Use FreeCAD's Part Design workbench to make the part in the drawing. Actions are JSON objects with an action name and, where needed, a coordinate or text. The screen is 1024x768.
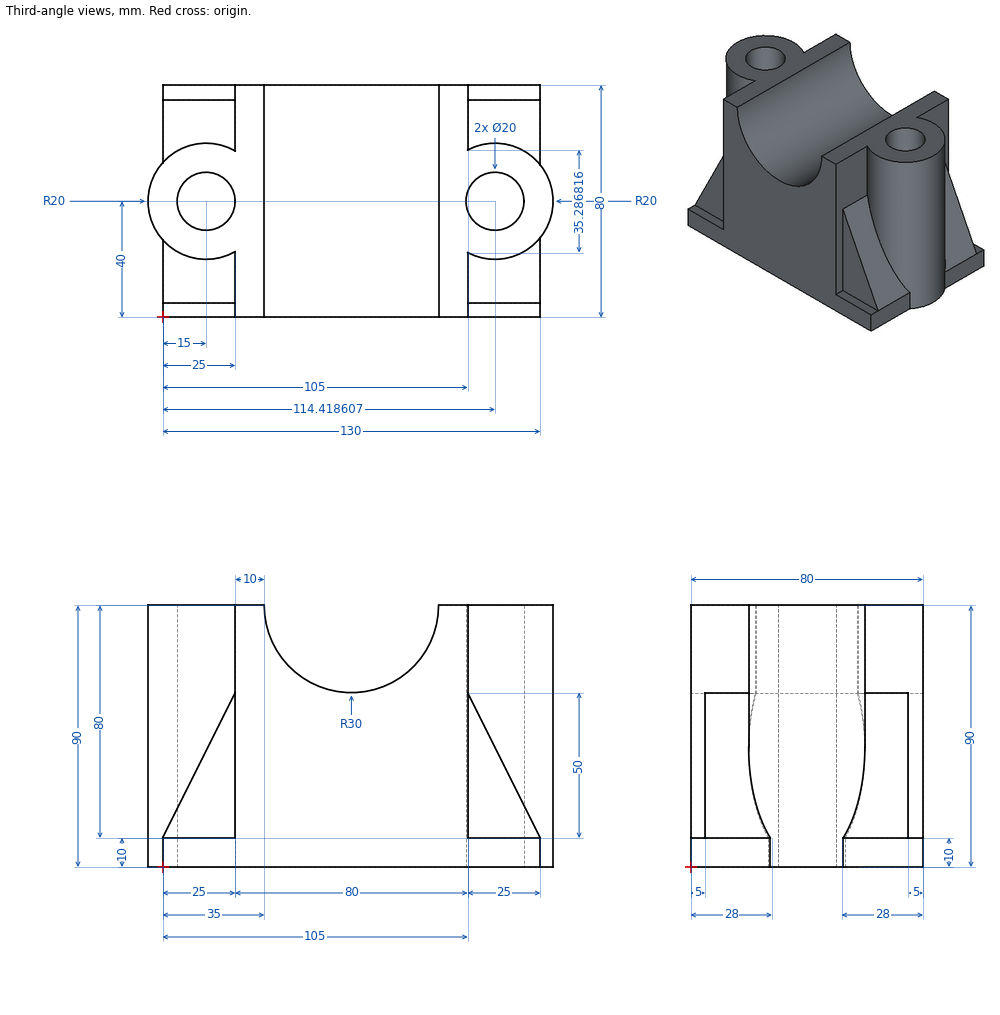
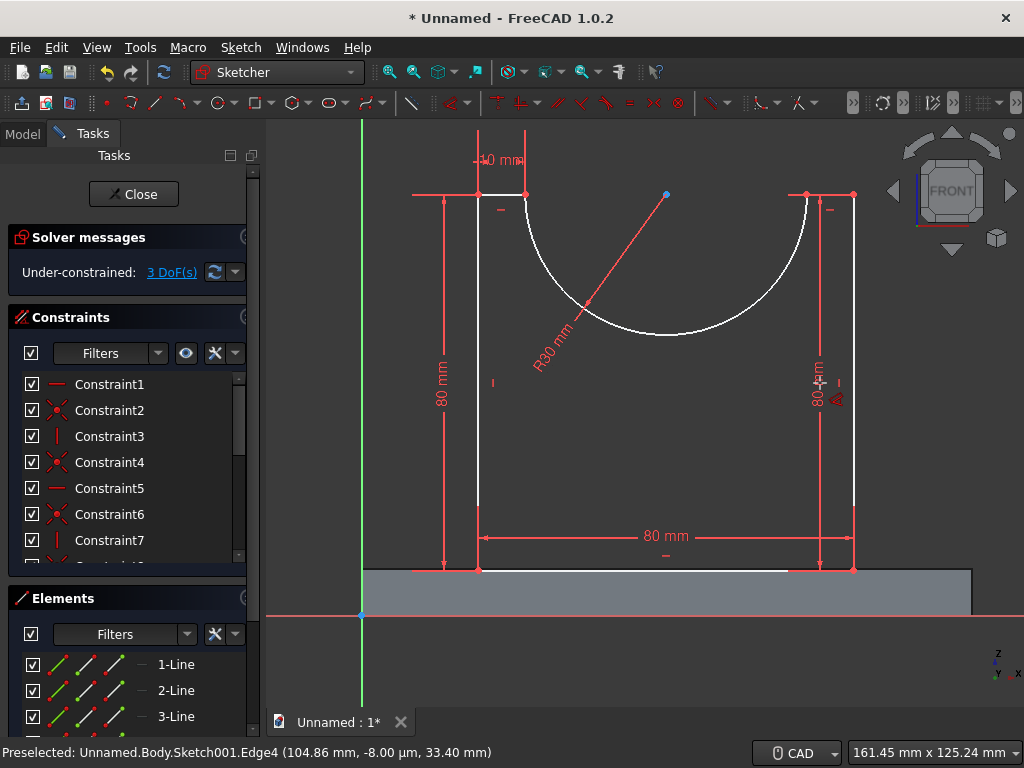
{"action": "left_click", "coordinate": [525, 195]}
{"action": "left_click", "coordinate": [443, 650]}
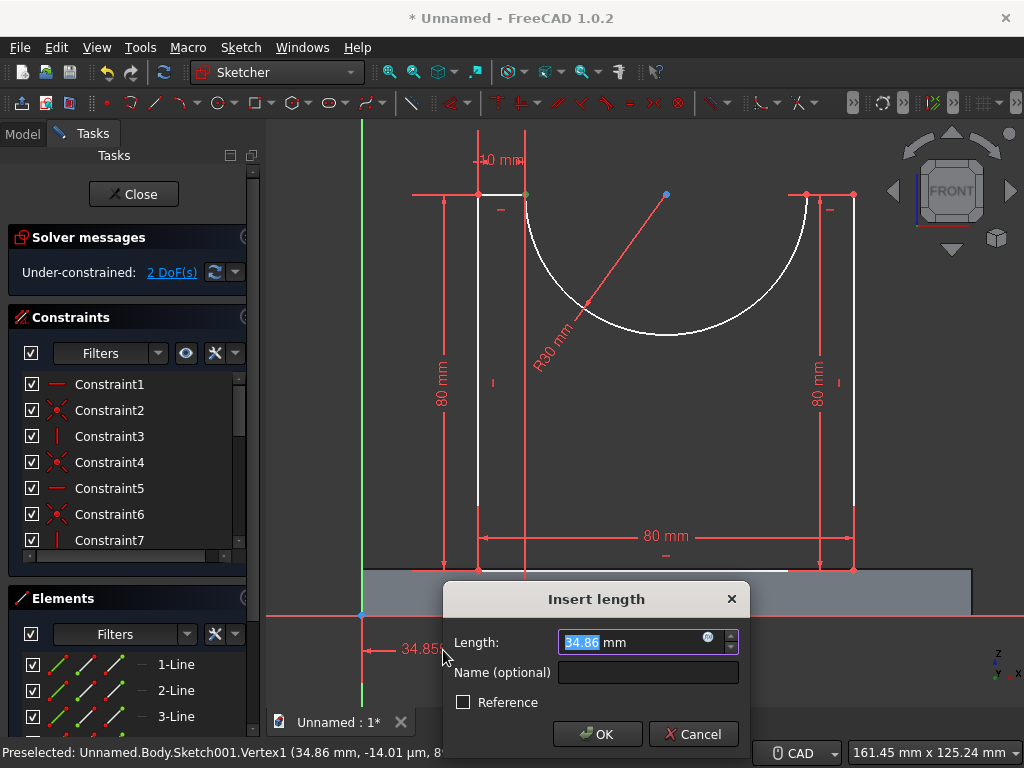
{"action": "type", "text": "35"}
{"action": "key", "text": "Return"}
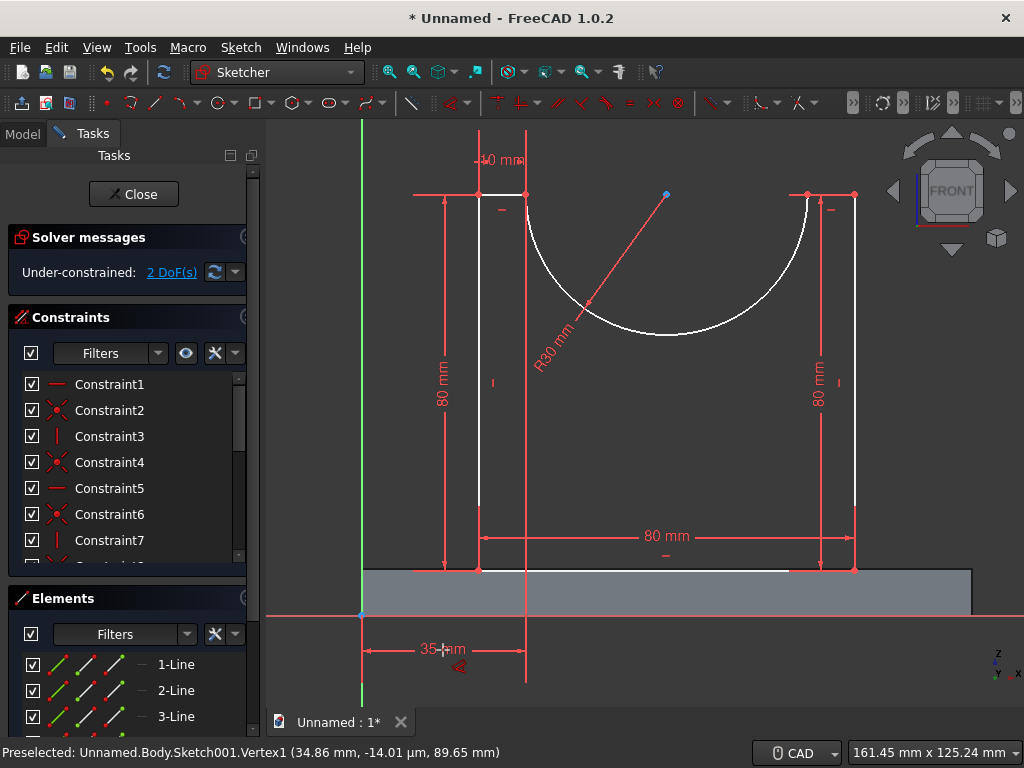
{"action": "left_click", "coordinate": [526, 195]}
{"action": "left_click", "coordinate": [328, 405]}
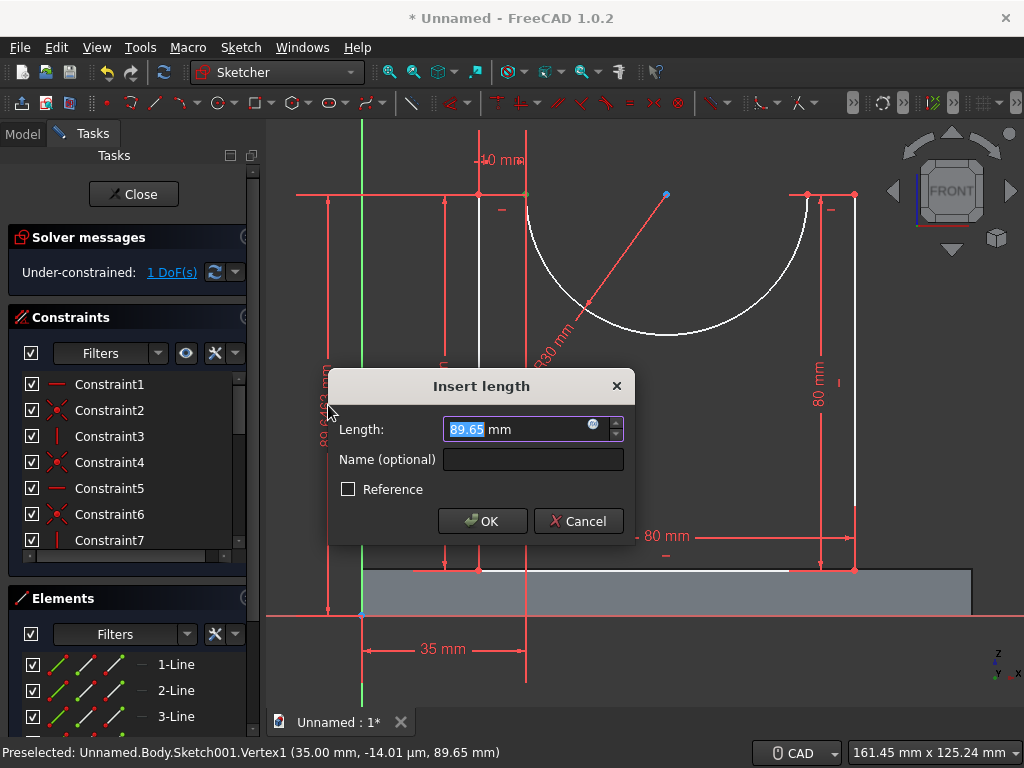
{"action": "type", "text": "90"}
{"action": "key", "text": "Return"}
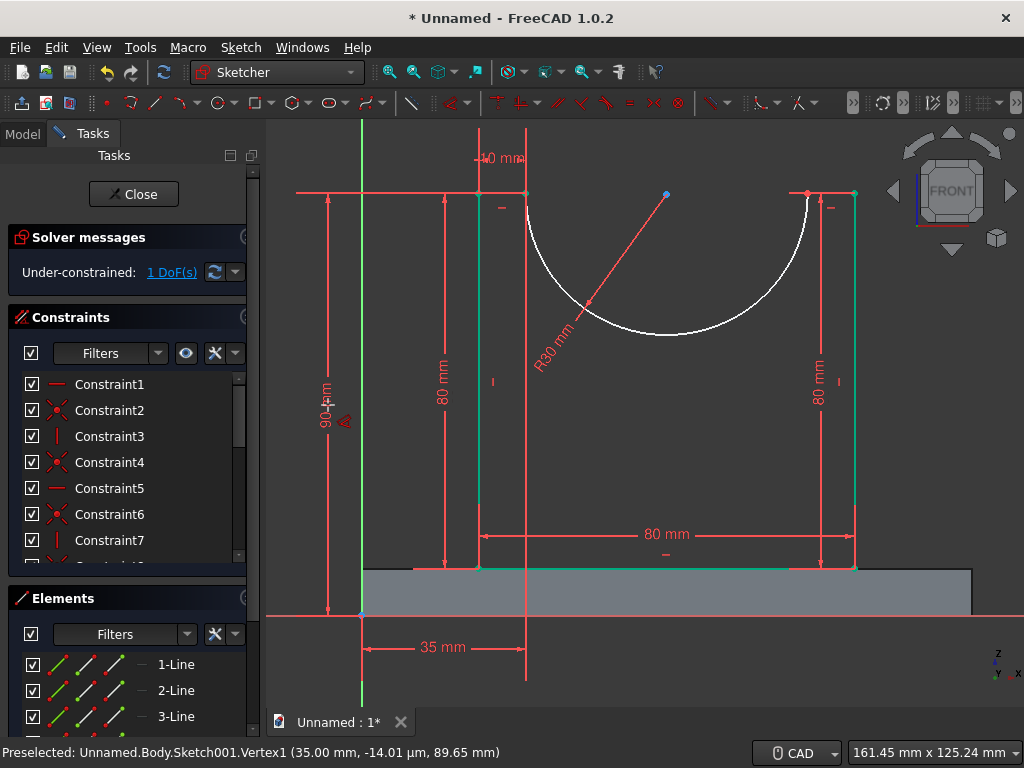
{"action": "left_click", "coordinate": [667, 194]}
{"action": "left_click", "coordinate": [328, 308]}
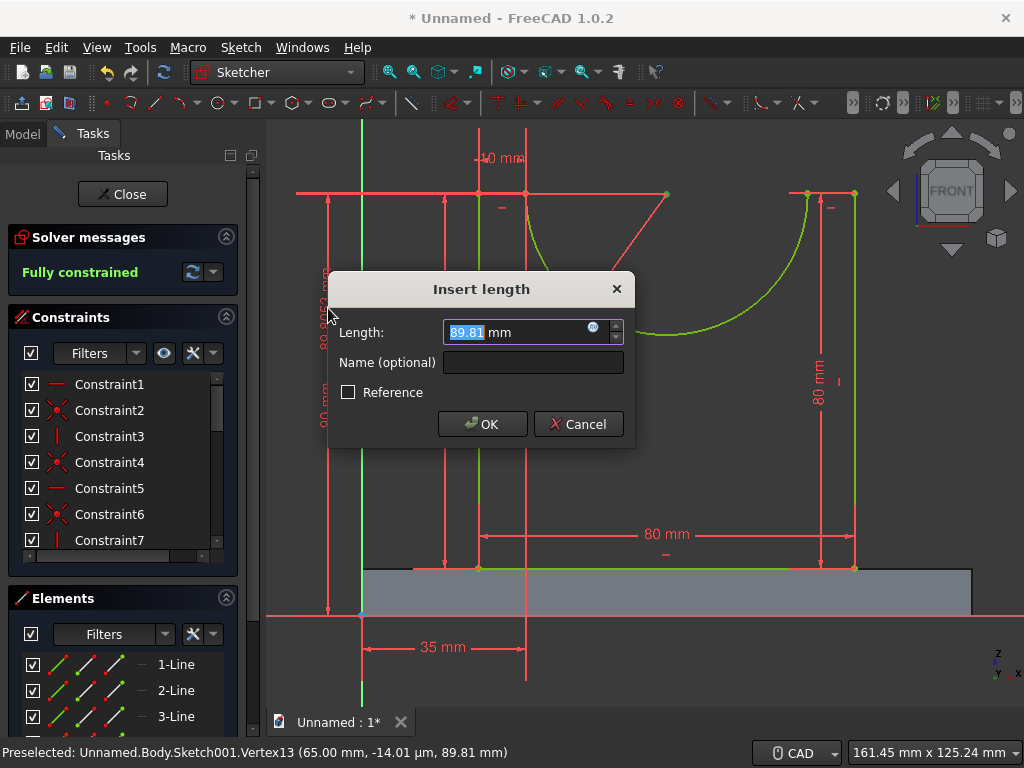
{"action": "type", "text": "90"}
{"action": "key", "text": "Return"}
{"action": "key", "text": "Escape"}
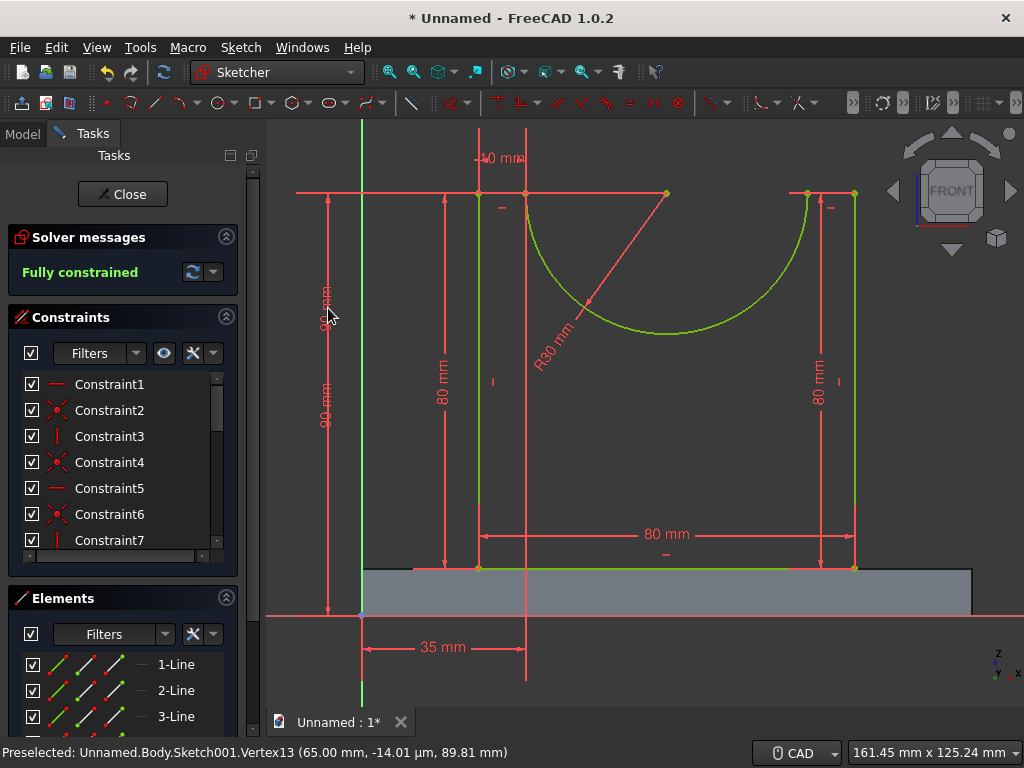
{"action": "left_click", "coordinate": [123, 194]}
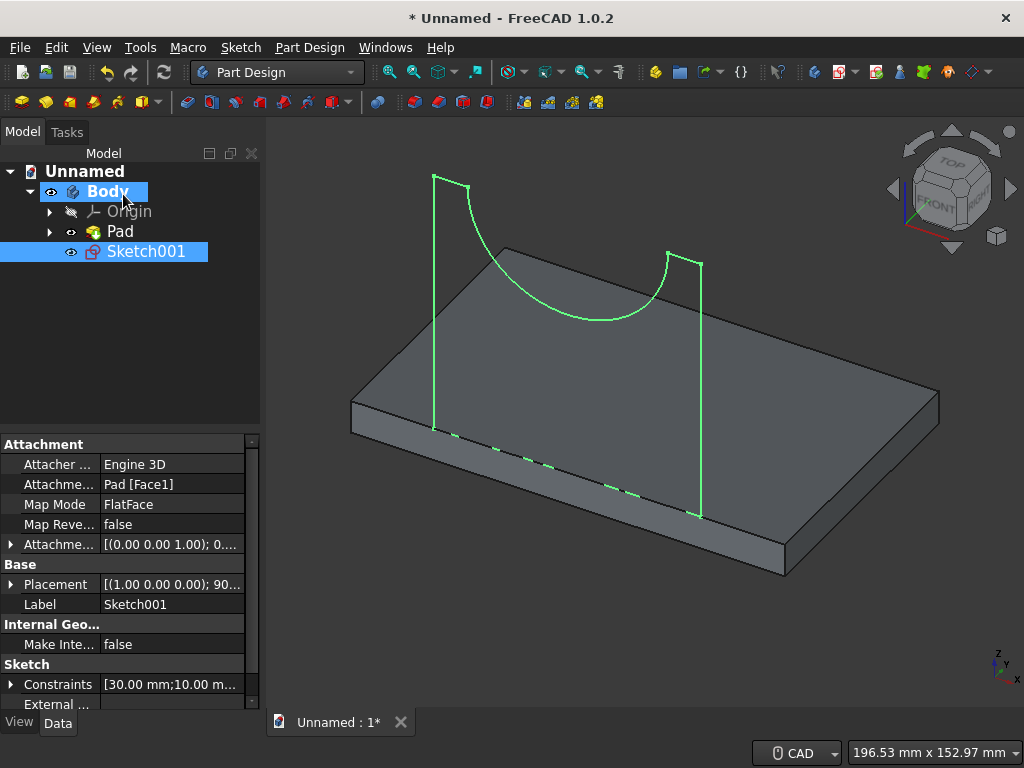
{"action": "left_click", "coordinate": [22, 102]}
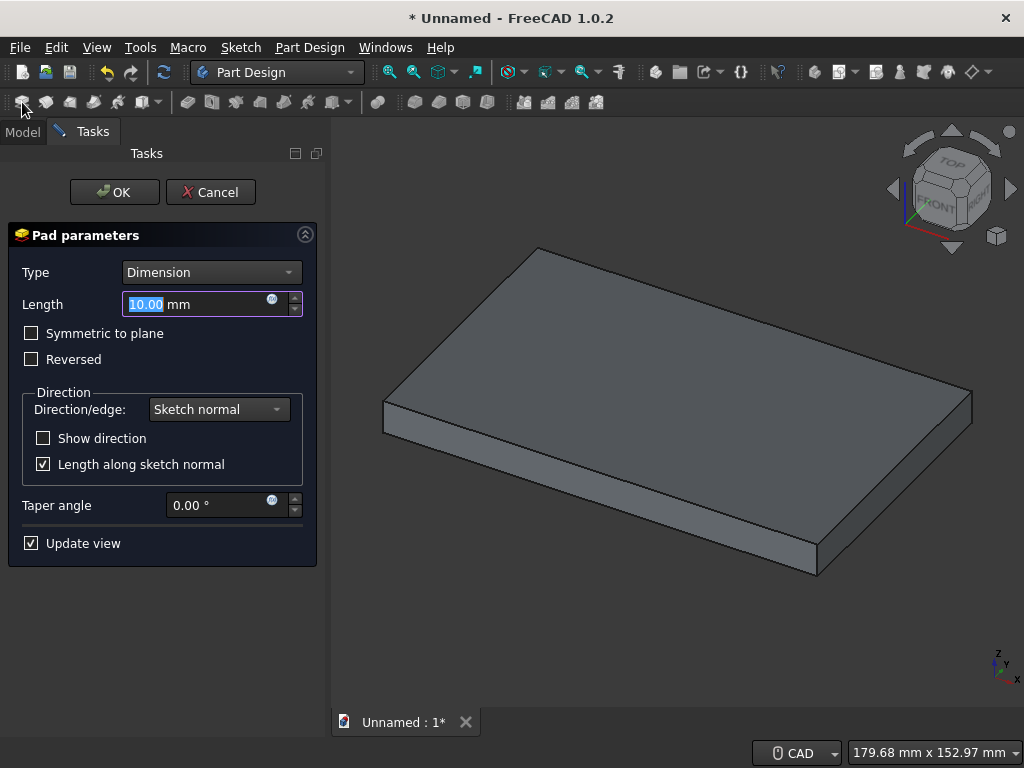
{"action": "type", "text": "80"}
{"action": "key", "text": "Tab"}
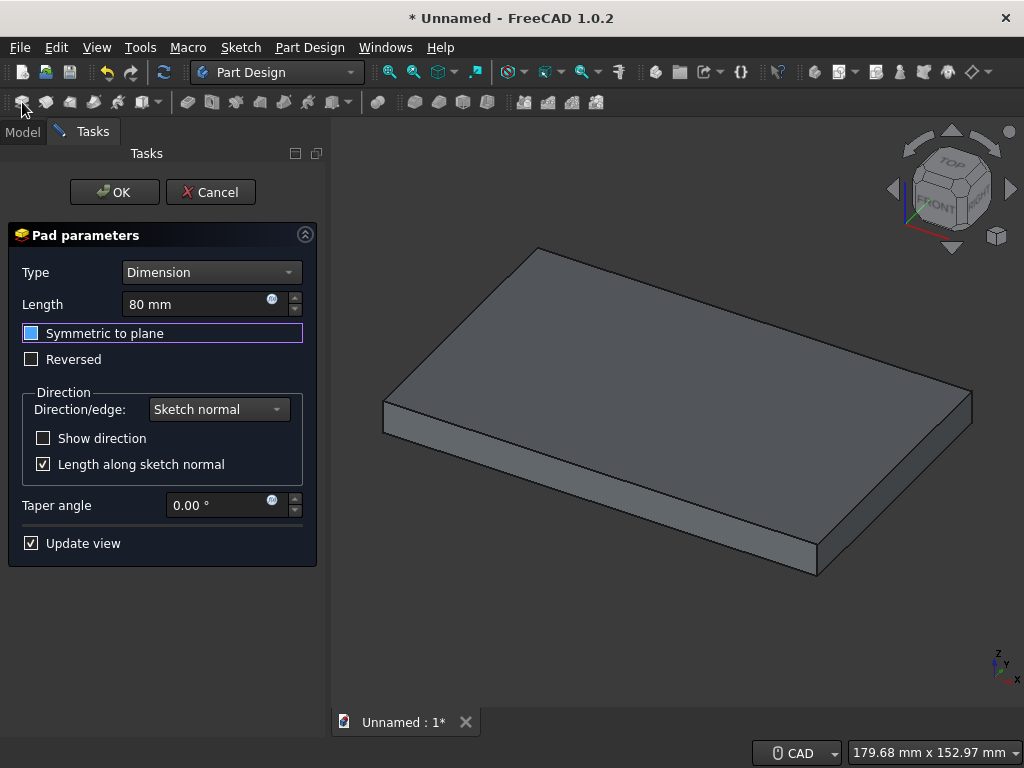
{"action": "left_click", "coordinate": [30, 359]}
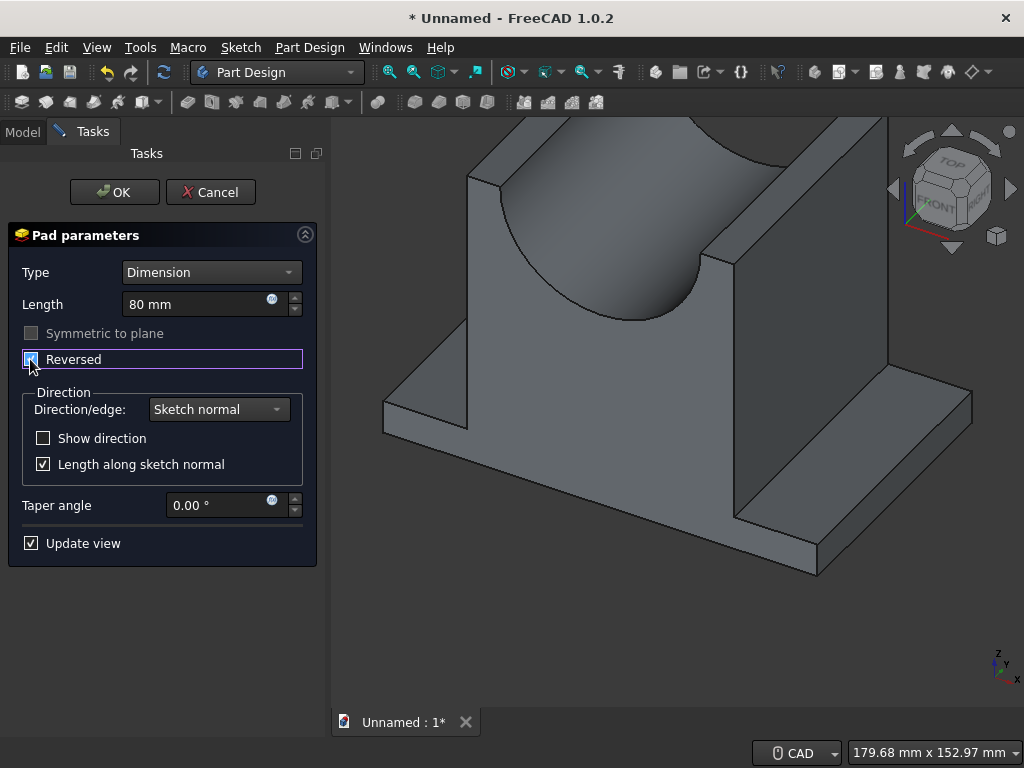
{"action": "left_click", "coordinate": [115, 192]}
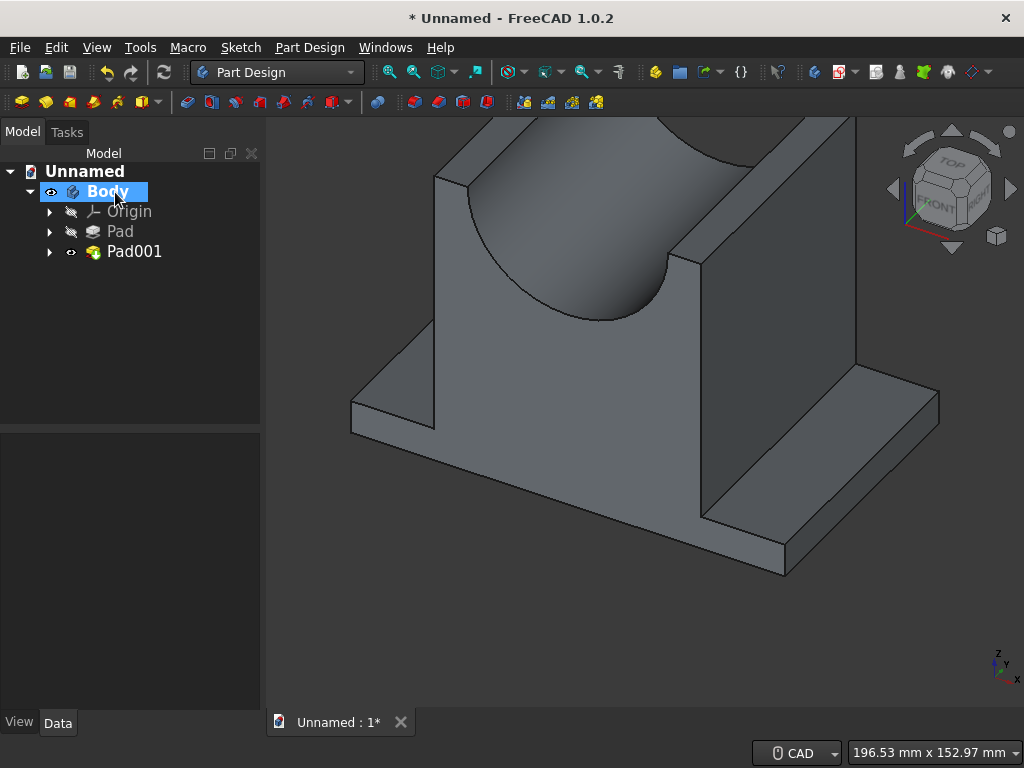
{"action": "left_click", "coordinate": [390, 72]}